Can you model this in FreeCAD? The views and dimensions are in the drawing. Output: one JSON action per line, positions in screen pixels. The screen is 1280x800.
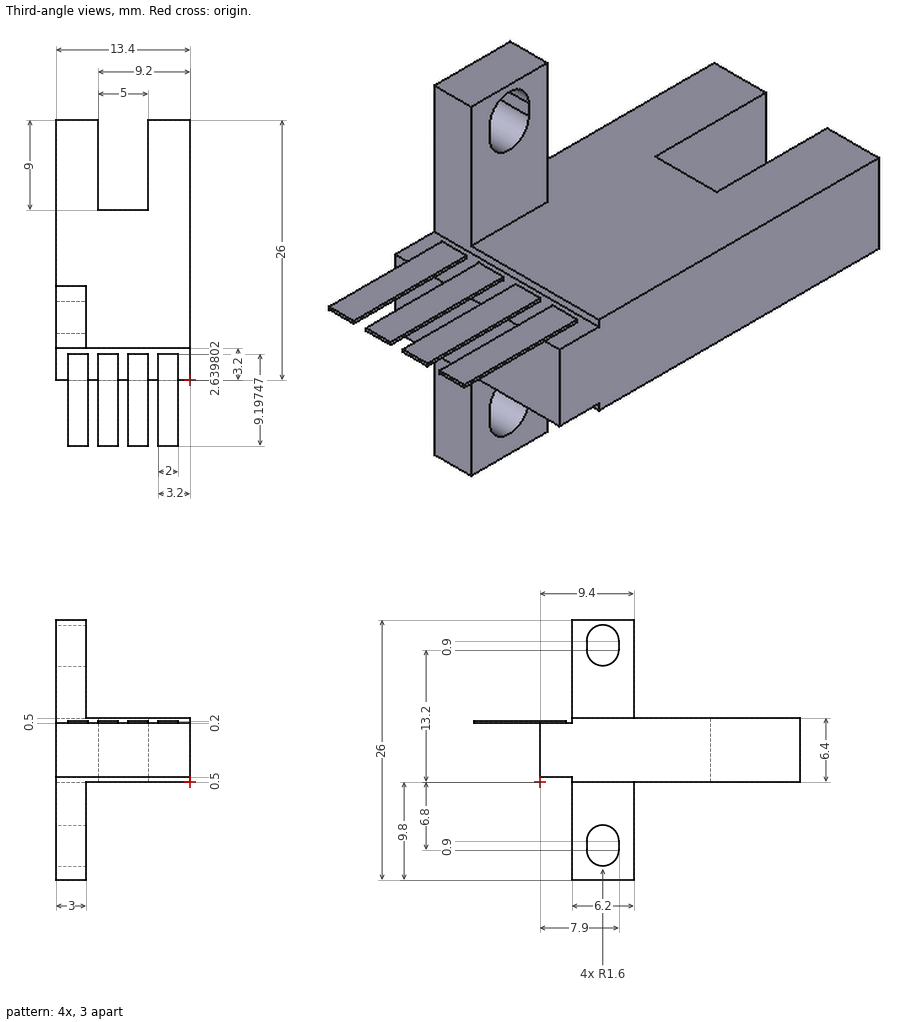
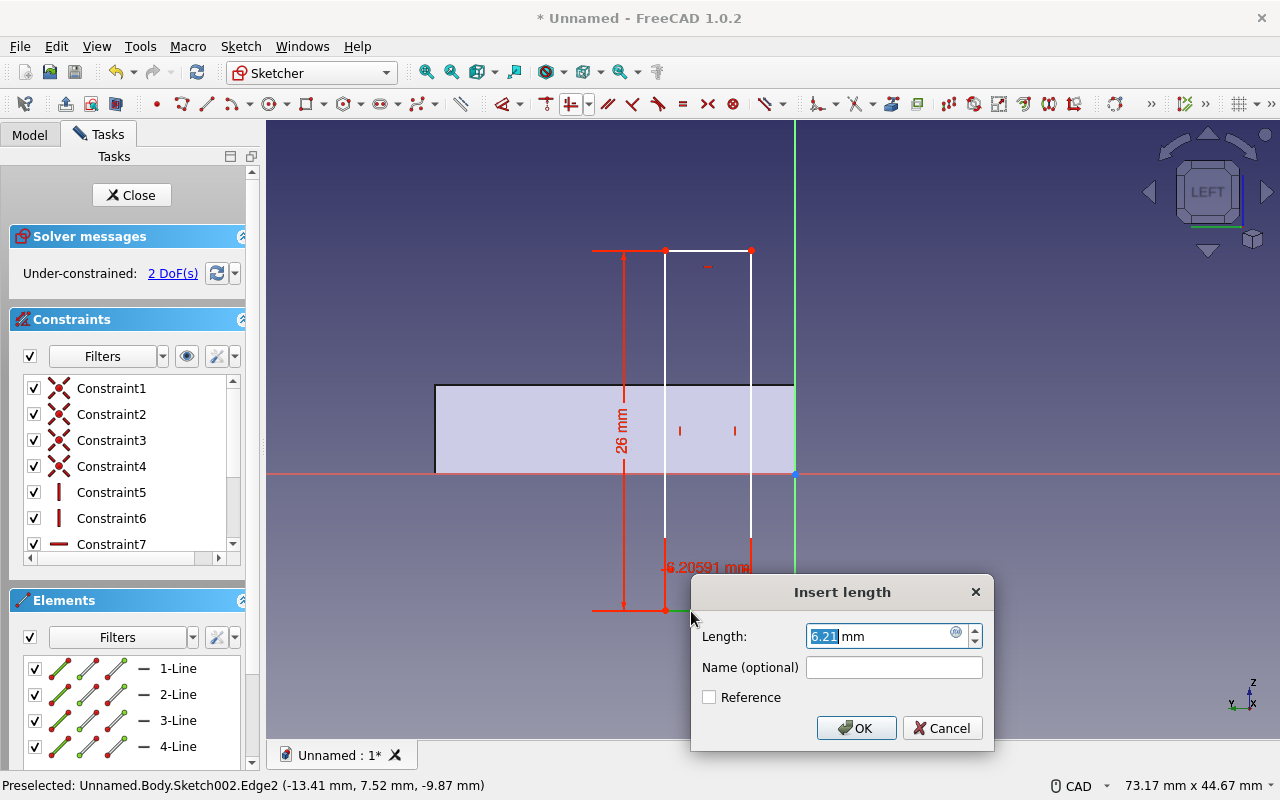
{"action": "type", "text": "6.2"}
{"action": "key", "text": "Return"}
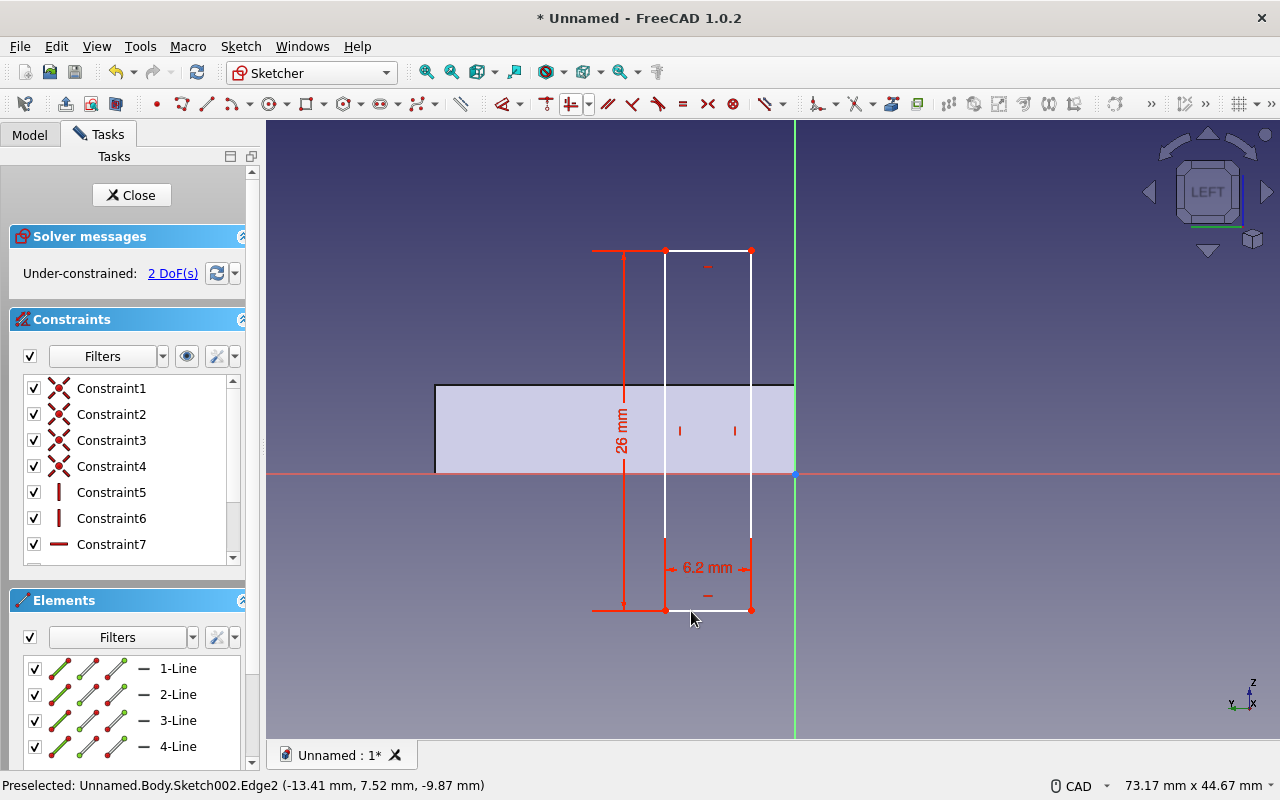
{"action": "left_click", "coordinate": [665, 251]}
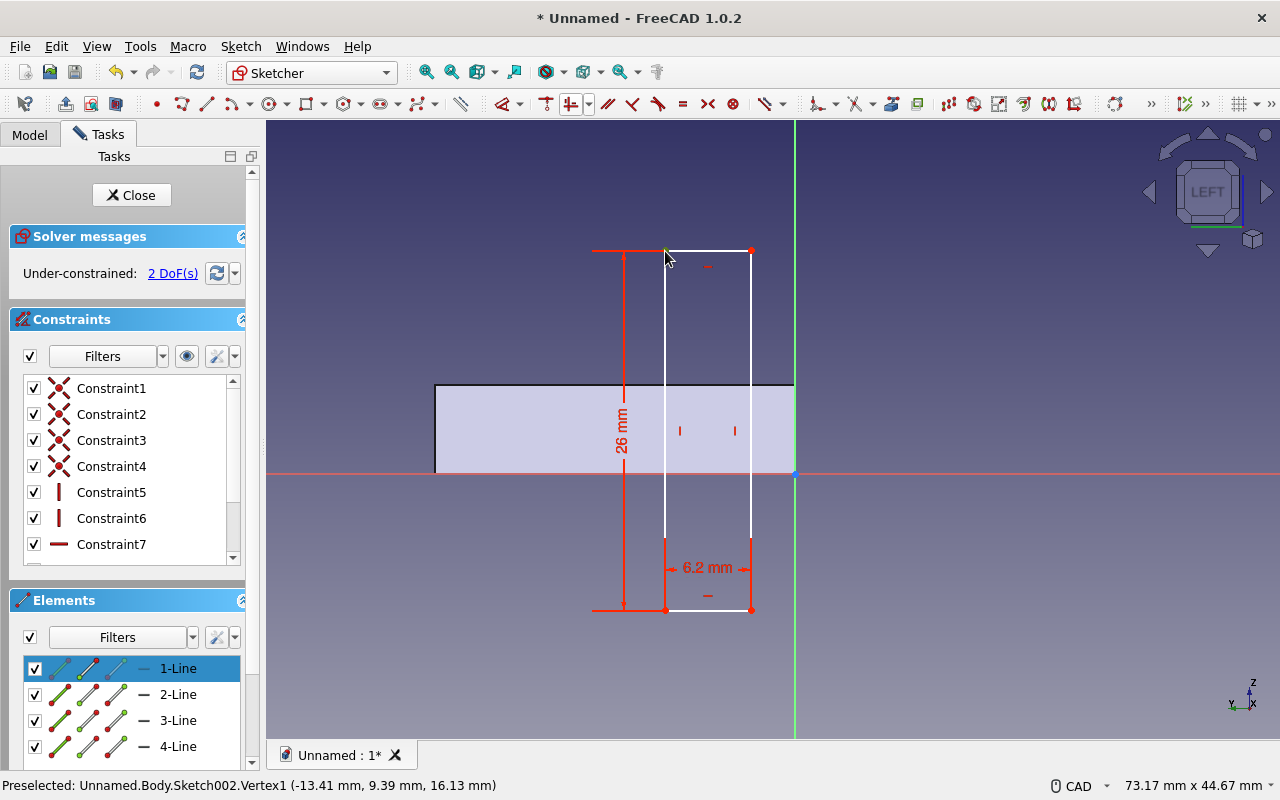
{"action": "left_click", "coordinate": [520, 104]}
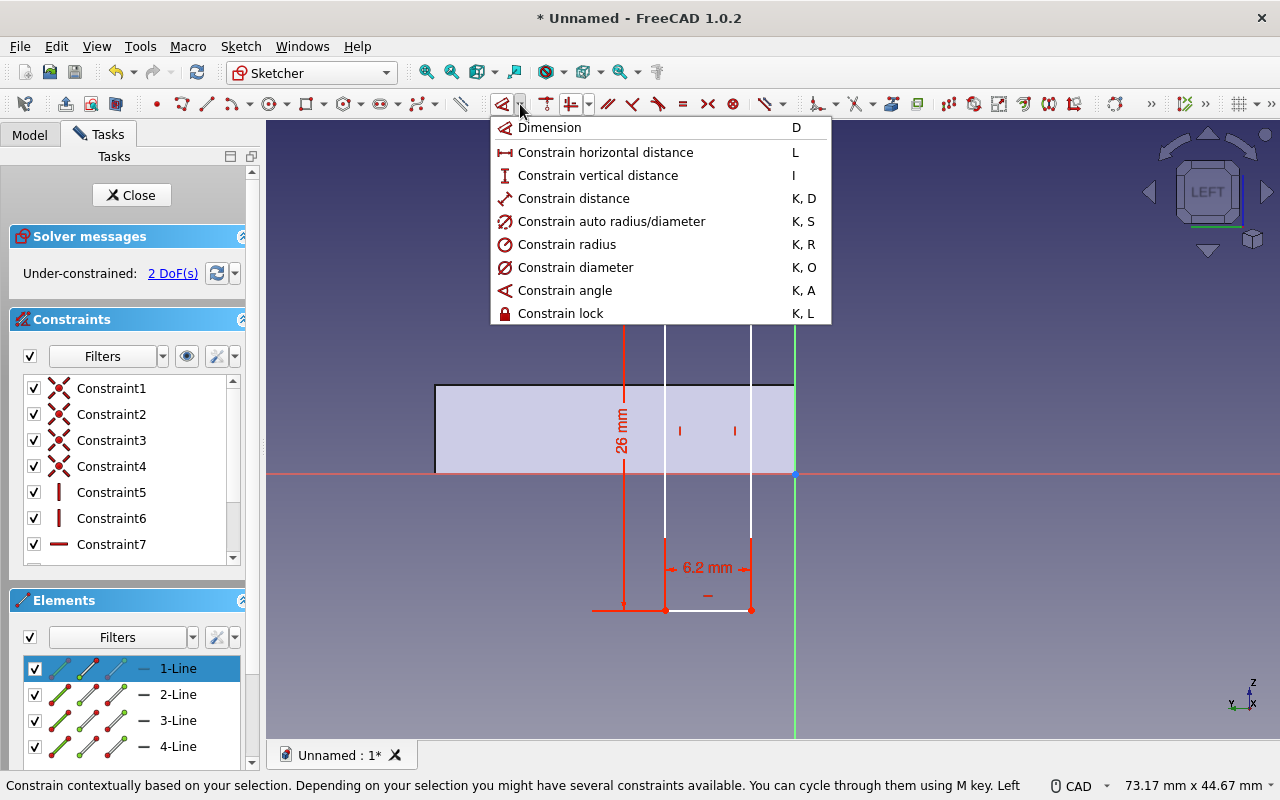
{"action": "left_click", "coordinate": [661, 152]}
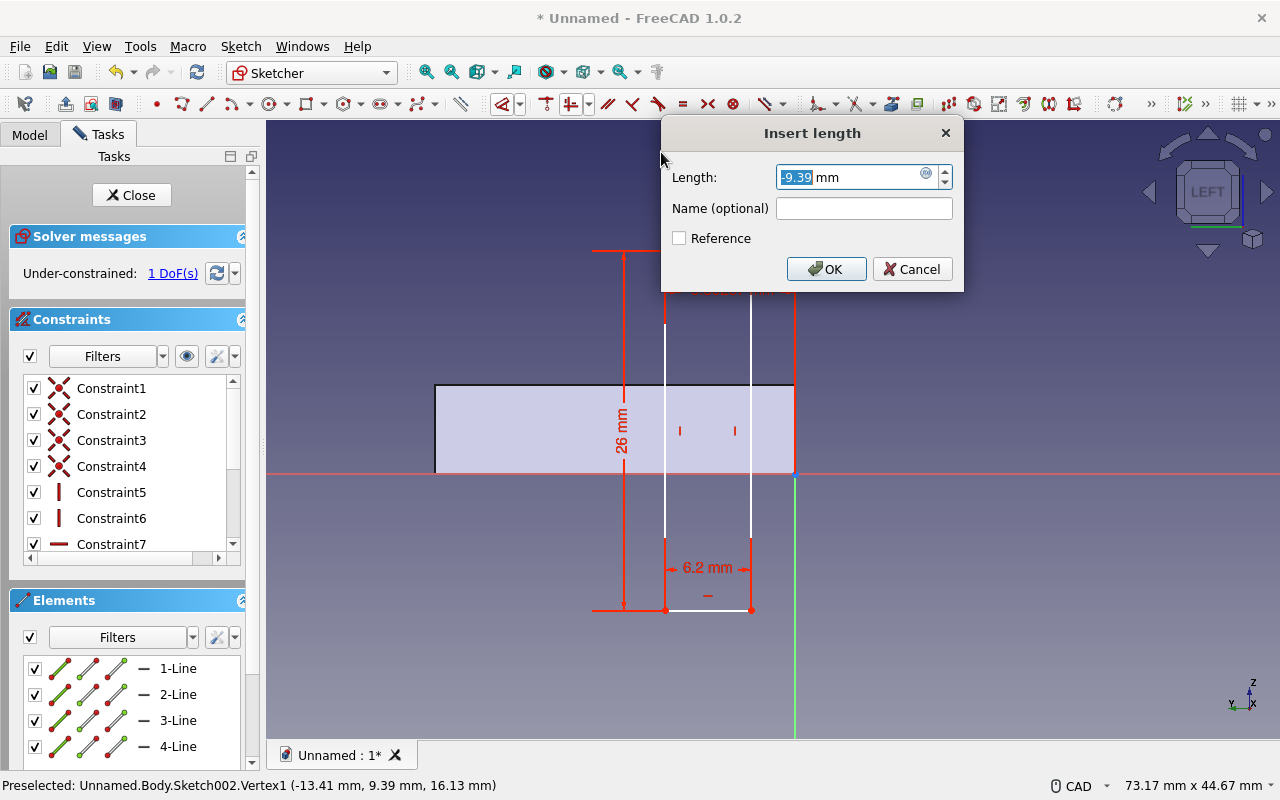
{"action": "type", "text": "-9.4"}
{"action": "key", "text": "Return"}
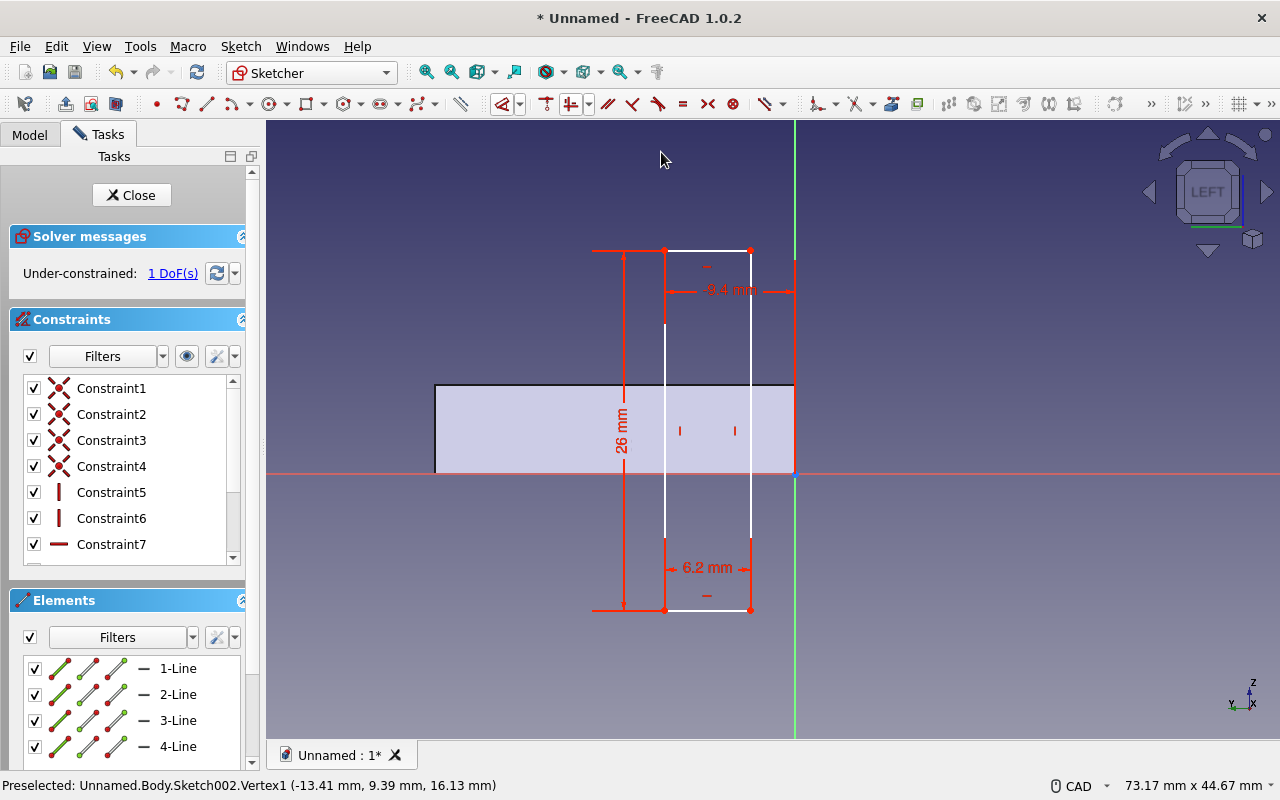
{"action": "left_click", "coordinate": [665, 611]}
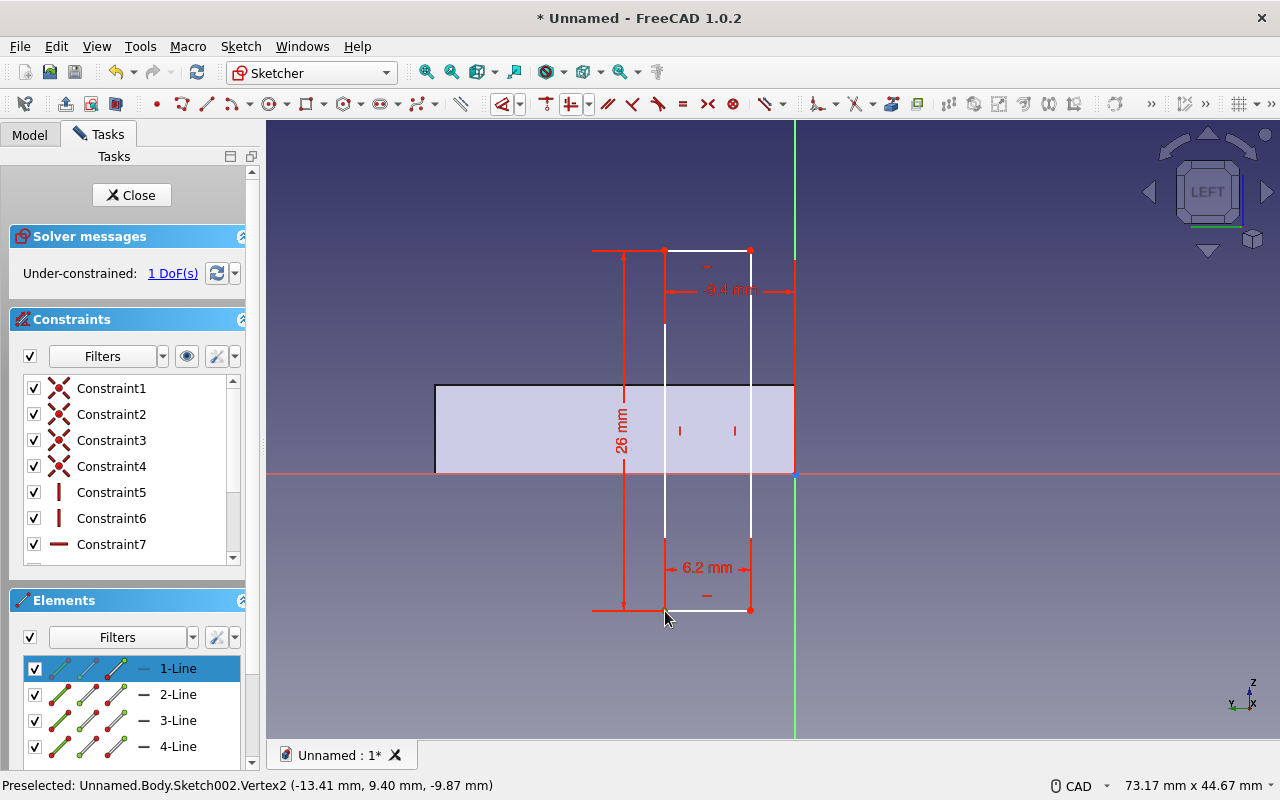
{"action": "key", "text": "i"}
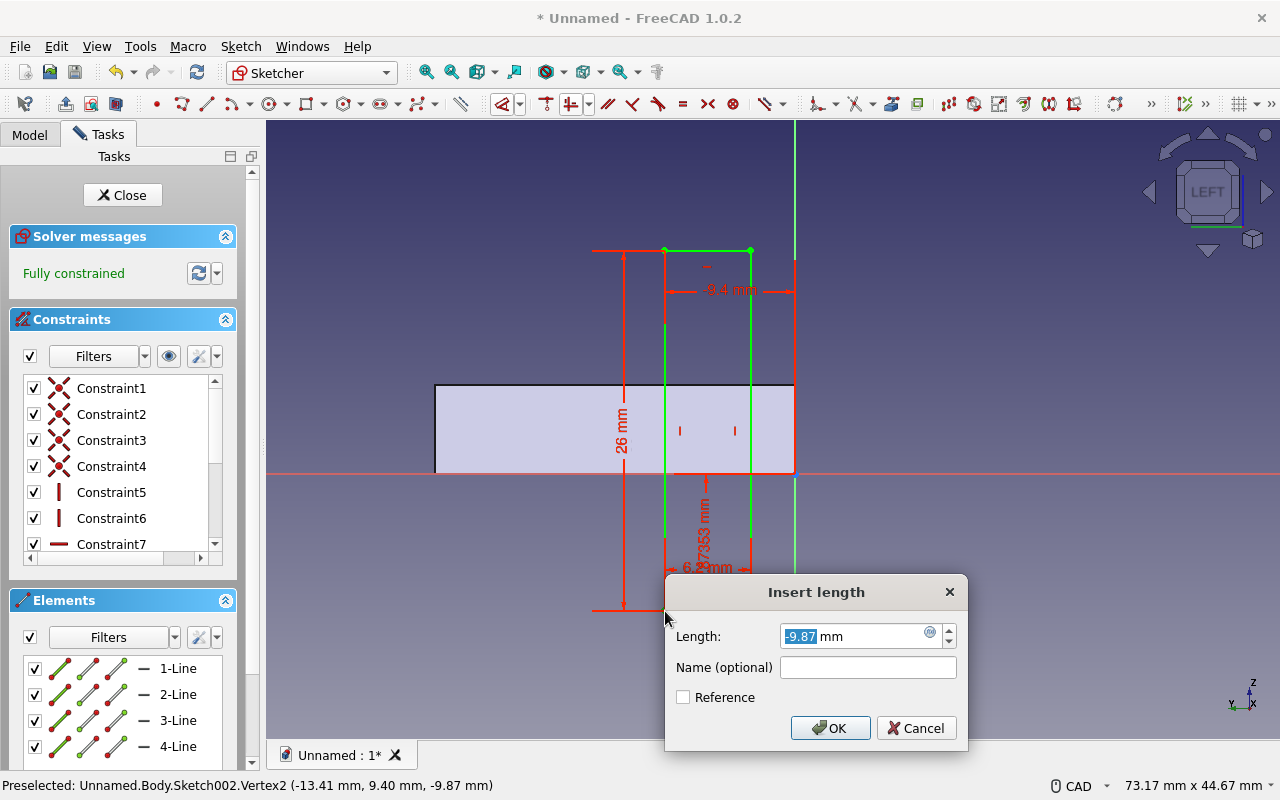
{"action": "type", "text": "-9.8"}
{"action": "key", "text": "Return"}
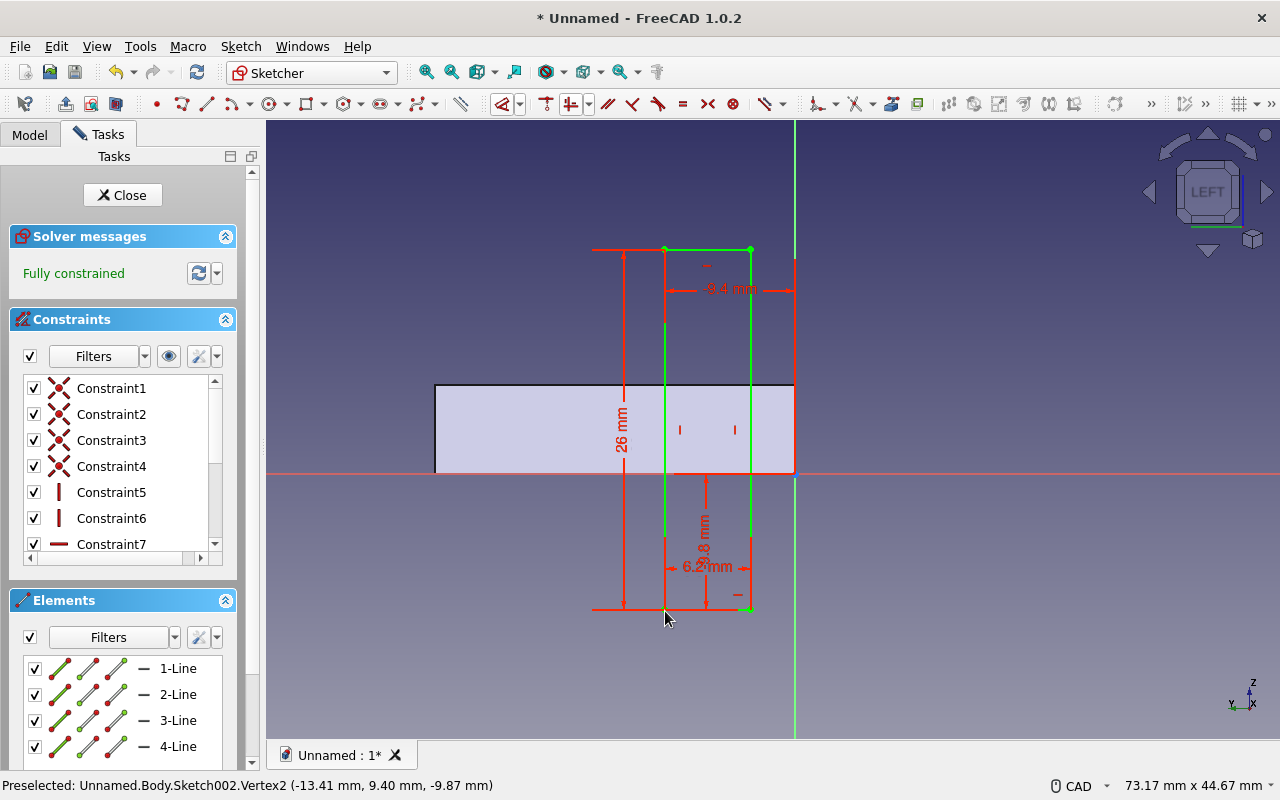
{"action": "left_click", "coordinate": [123, 195]}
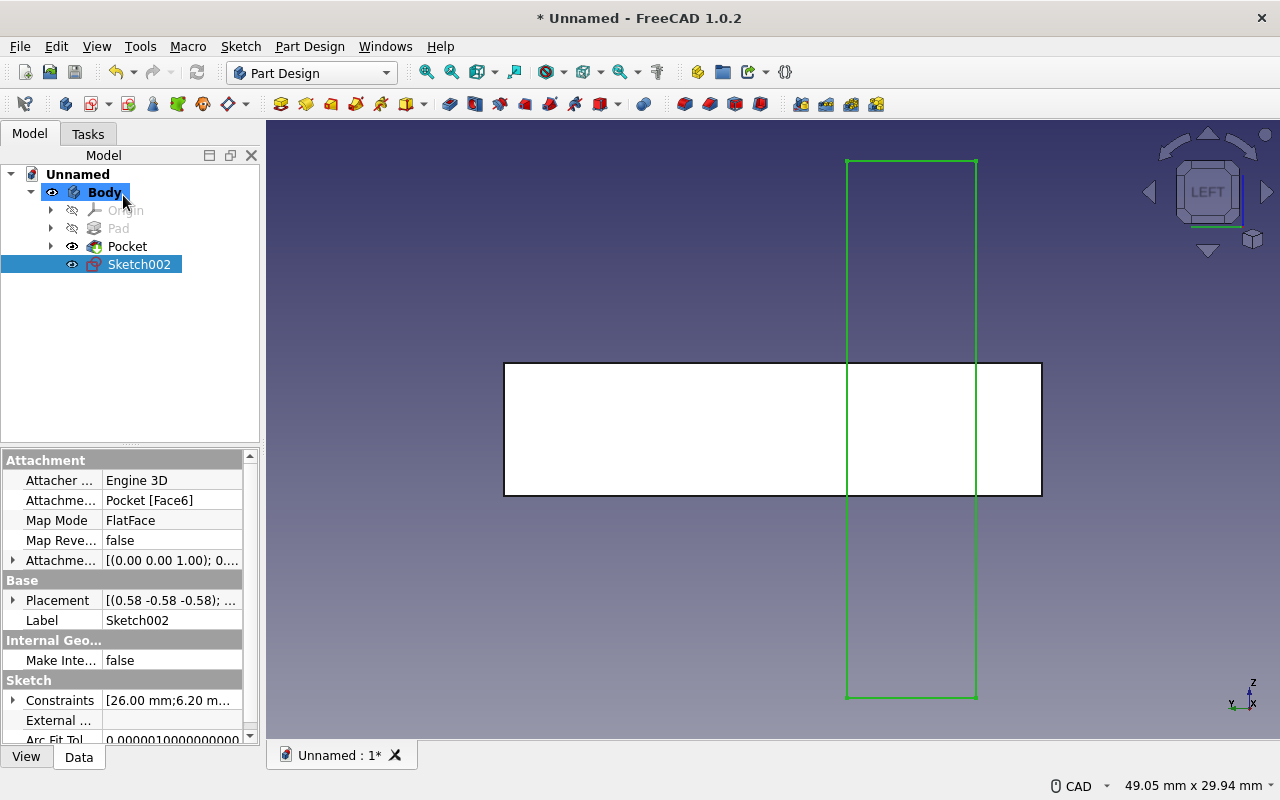
{"action": "left_click", "coordinate": [281, 104]}